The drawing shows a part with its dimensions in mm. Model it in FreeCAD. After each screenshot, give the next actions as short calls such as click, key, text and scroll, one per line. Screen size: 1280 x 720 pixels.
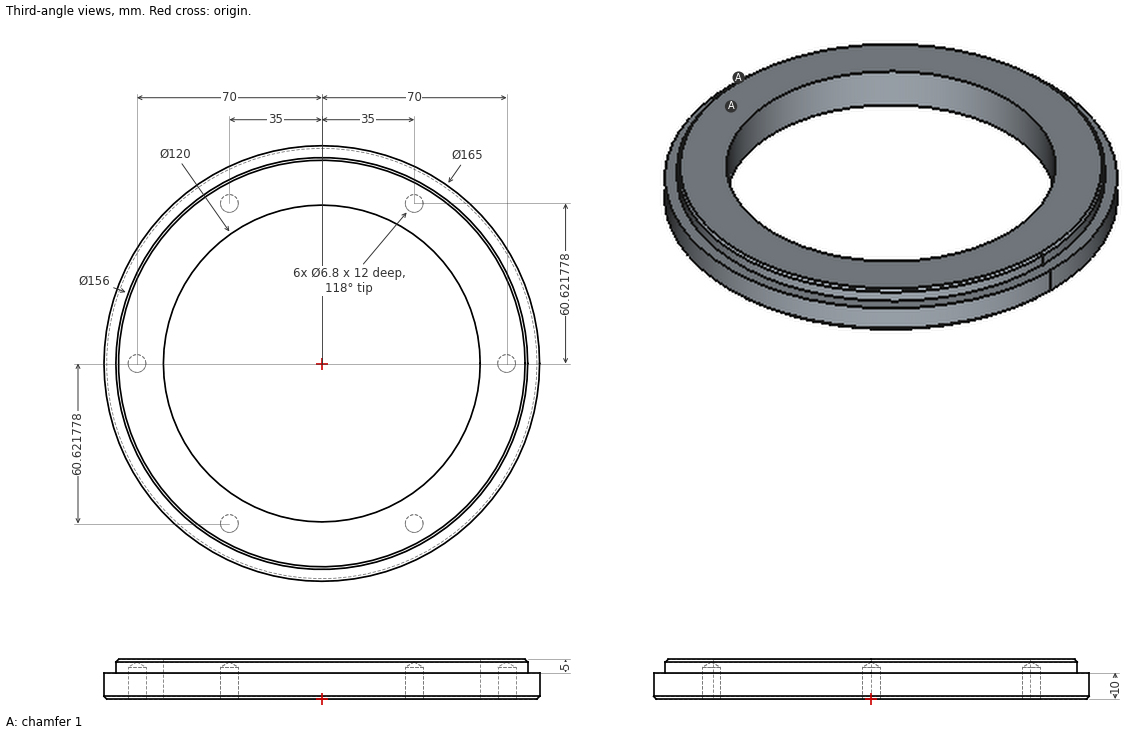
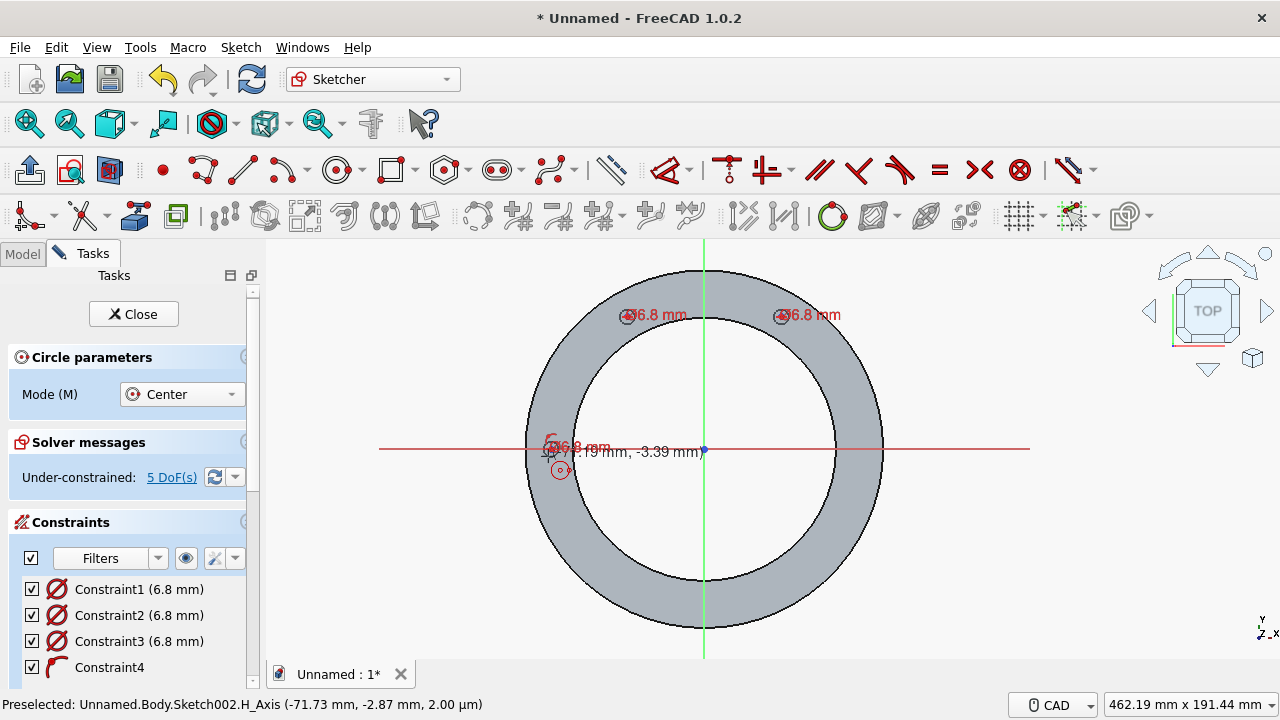
scroll(628, 582, up, 6)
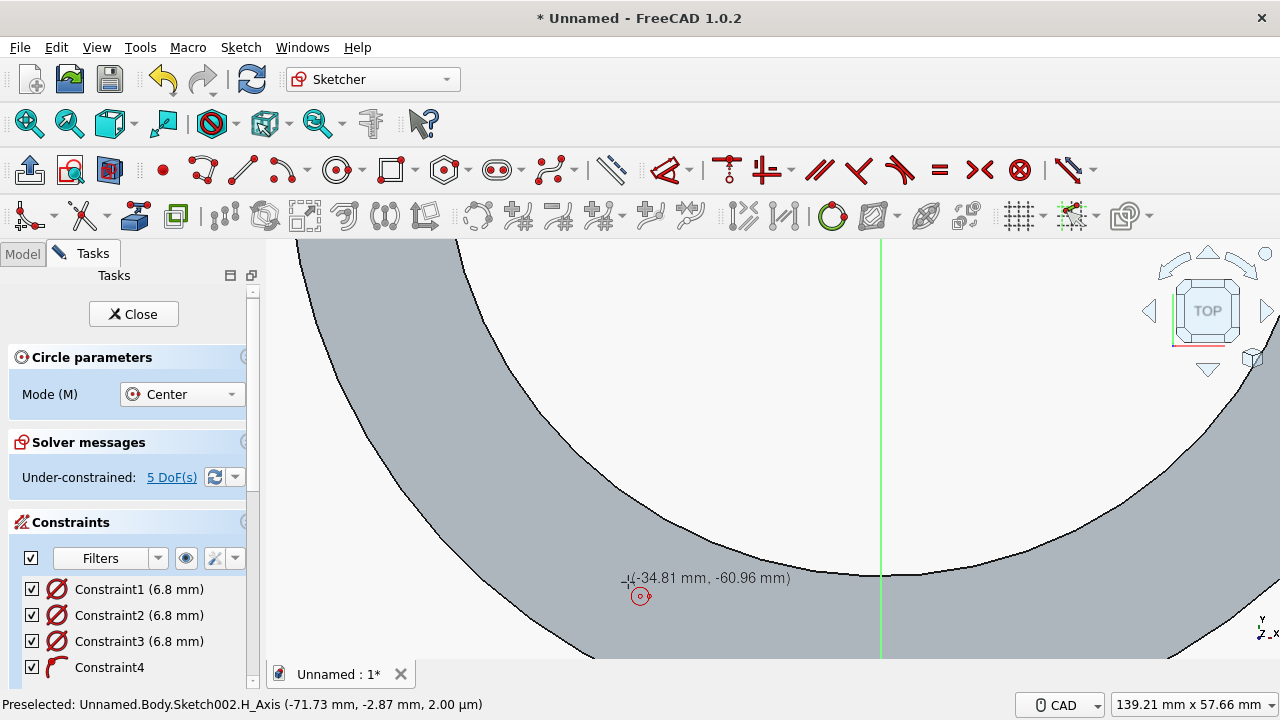
scroll(629, 582, down, 6)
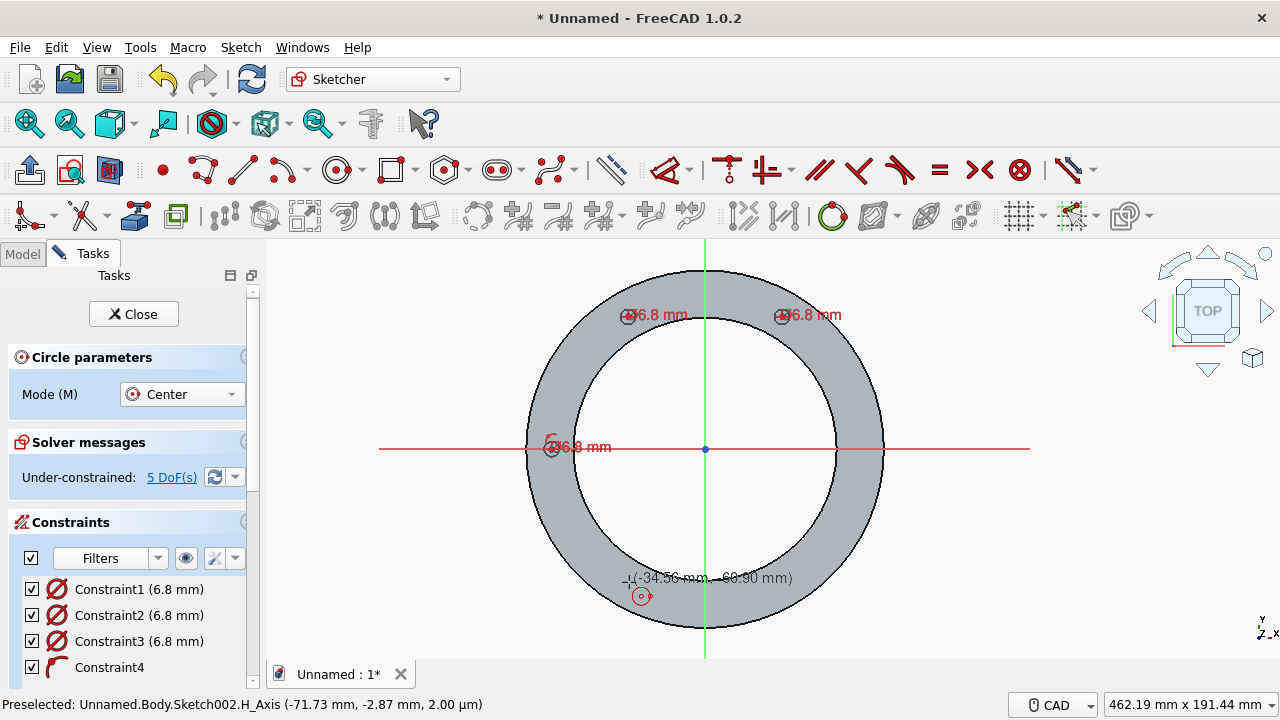
click(628, 582)
move(634, 577)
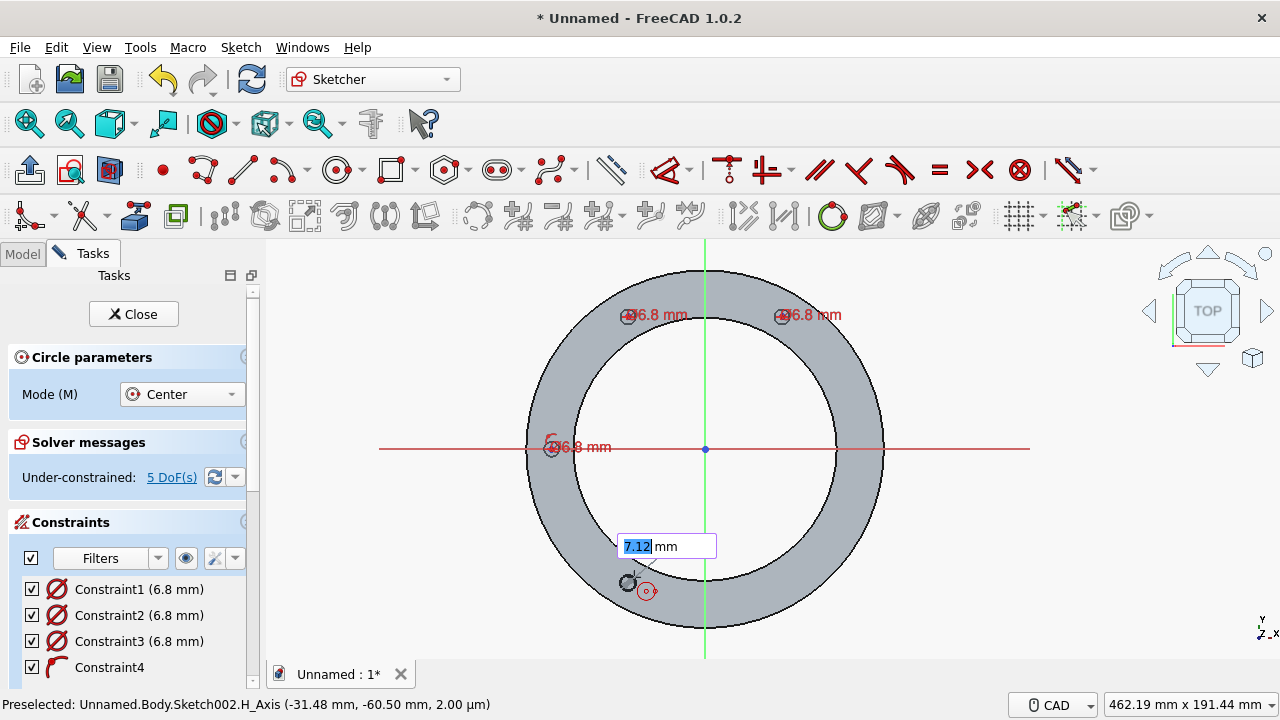
text(6.8)
key(Return)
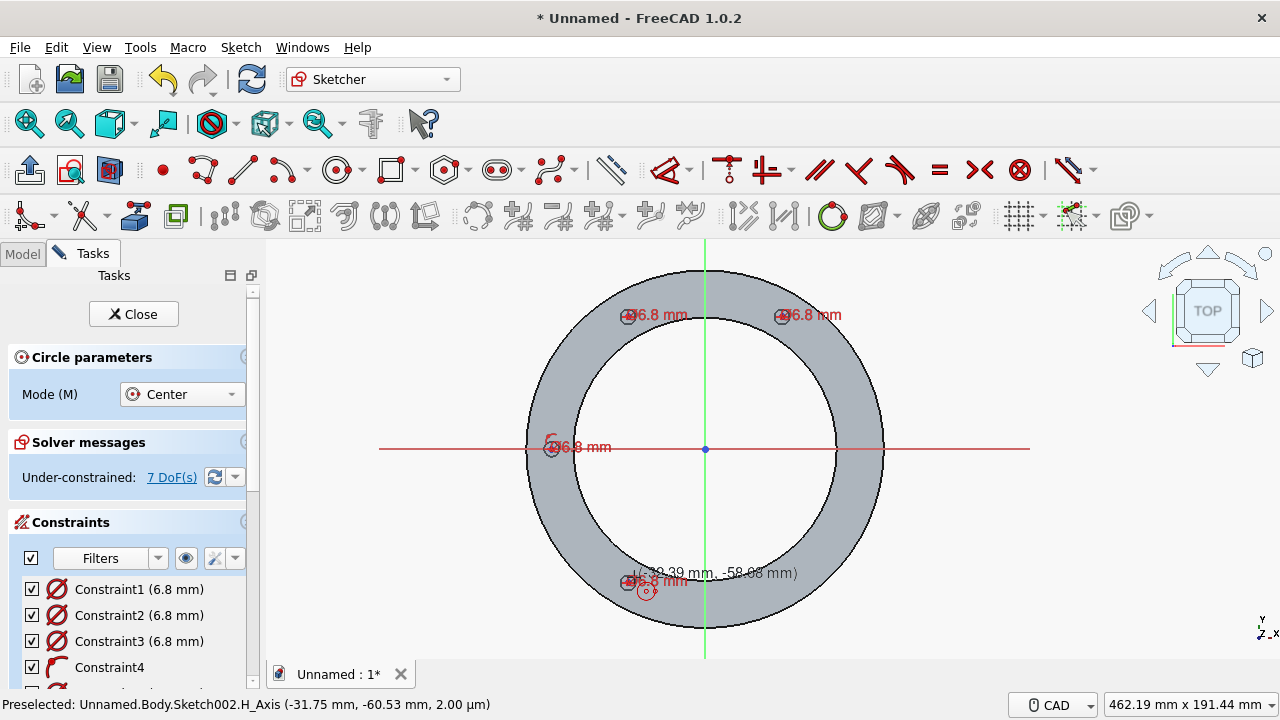
scroll(782, 582, up, 6)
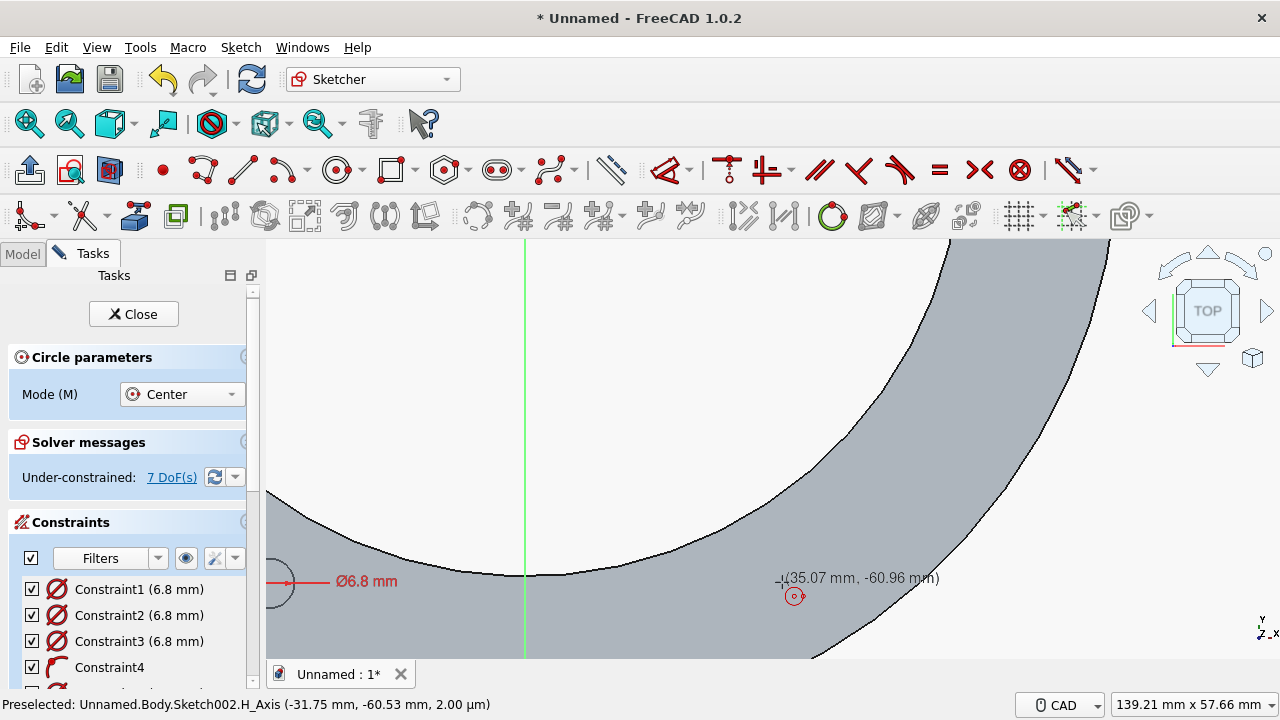
scroll(782, 582, down, 6)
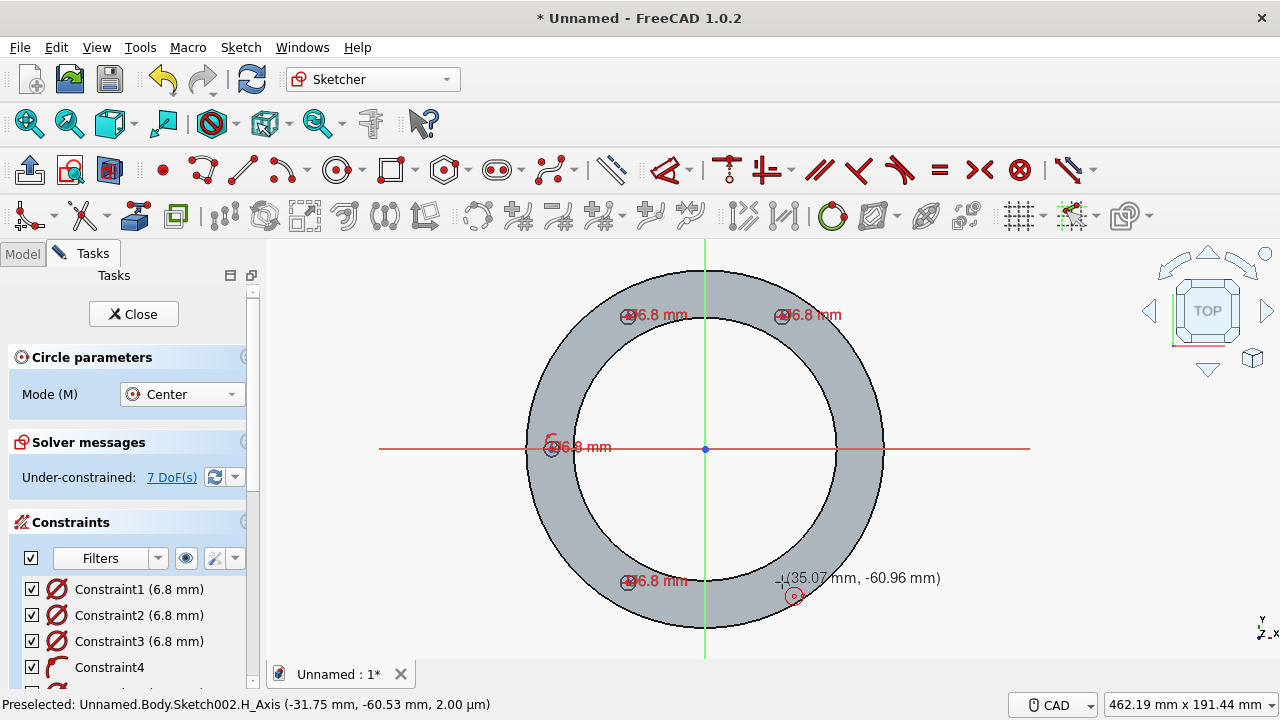
click(782, 582)
move(787, 577)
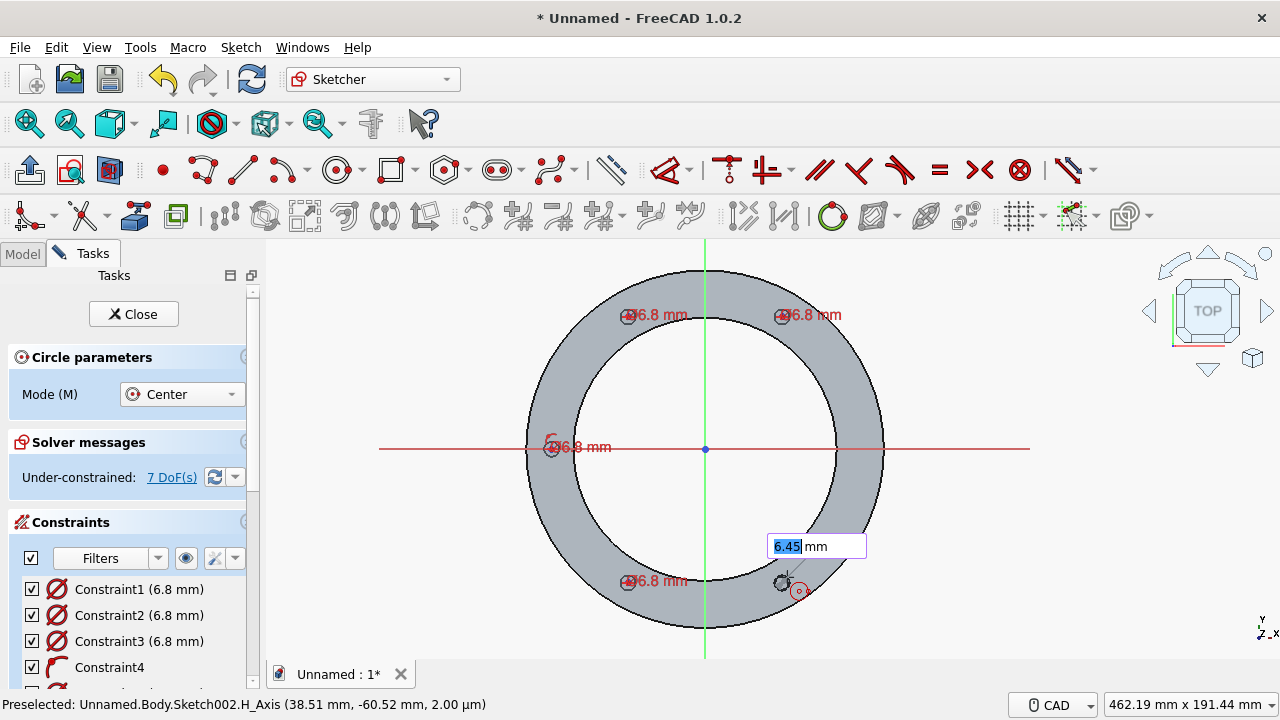
text(6.8)
key(Return)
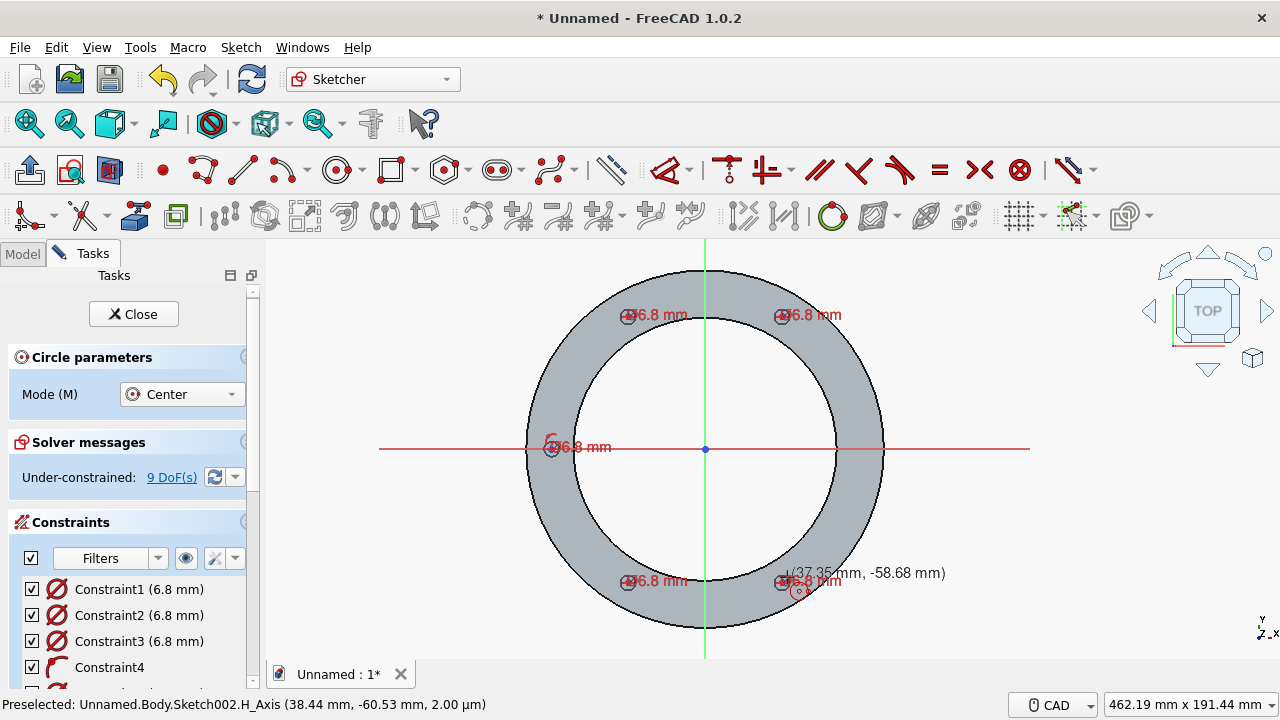
scroll(859, 449, up, 6)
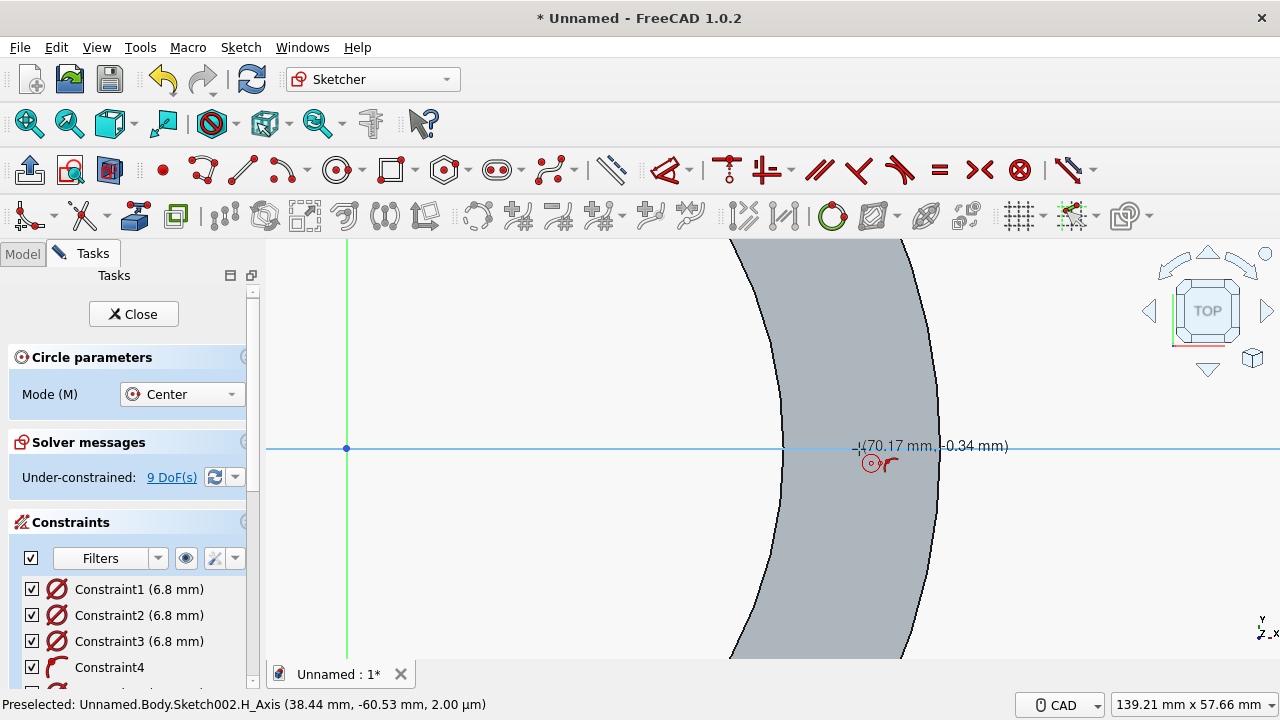
scroll(859, 449, down, 6)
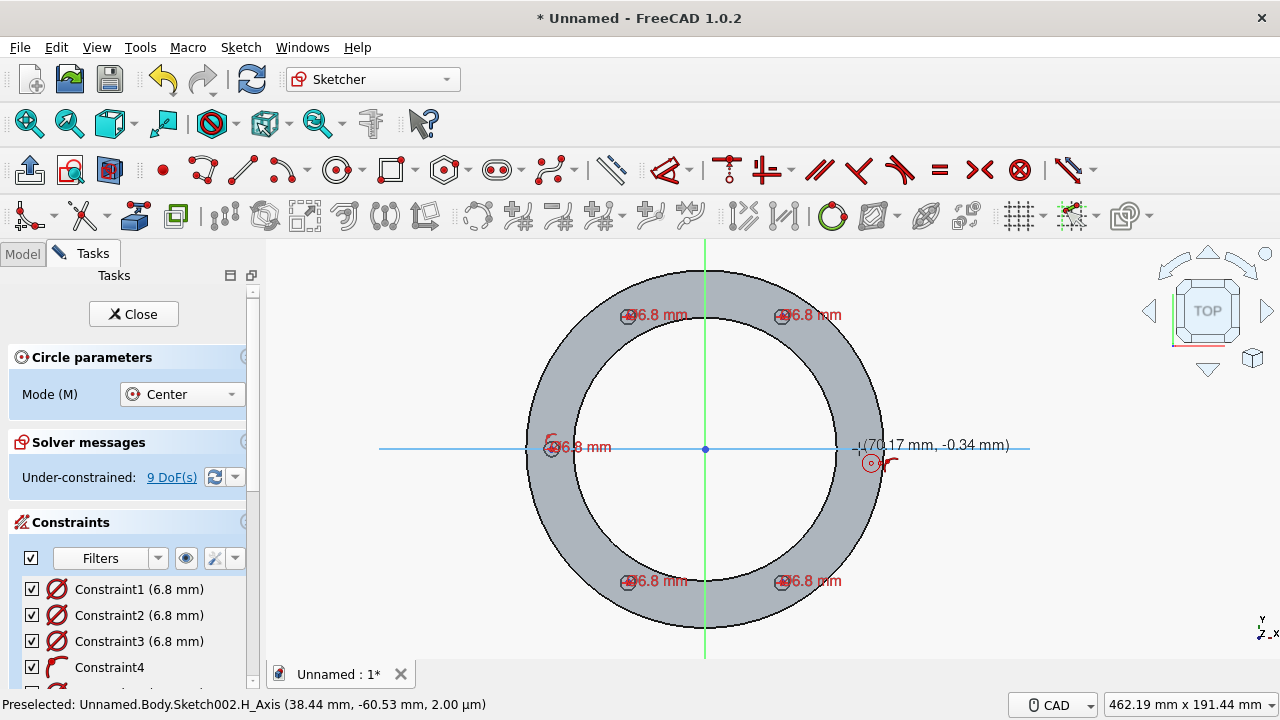
click(859, 449)